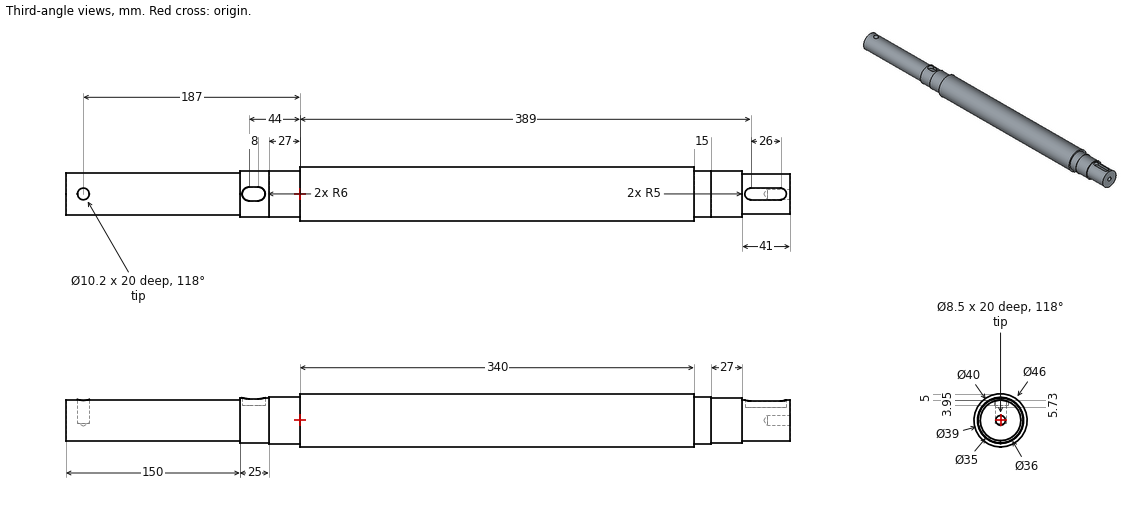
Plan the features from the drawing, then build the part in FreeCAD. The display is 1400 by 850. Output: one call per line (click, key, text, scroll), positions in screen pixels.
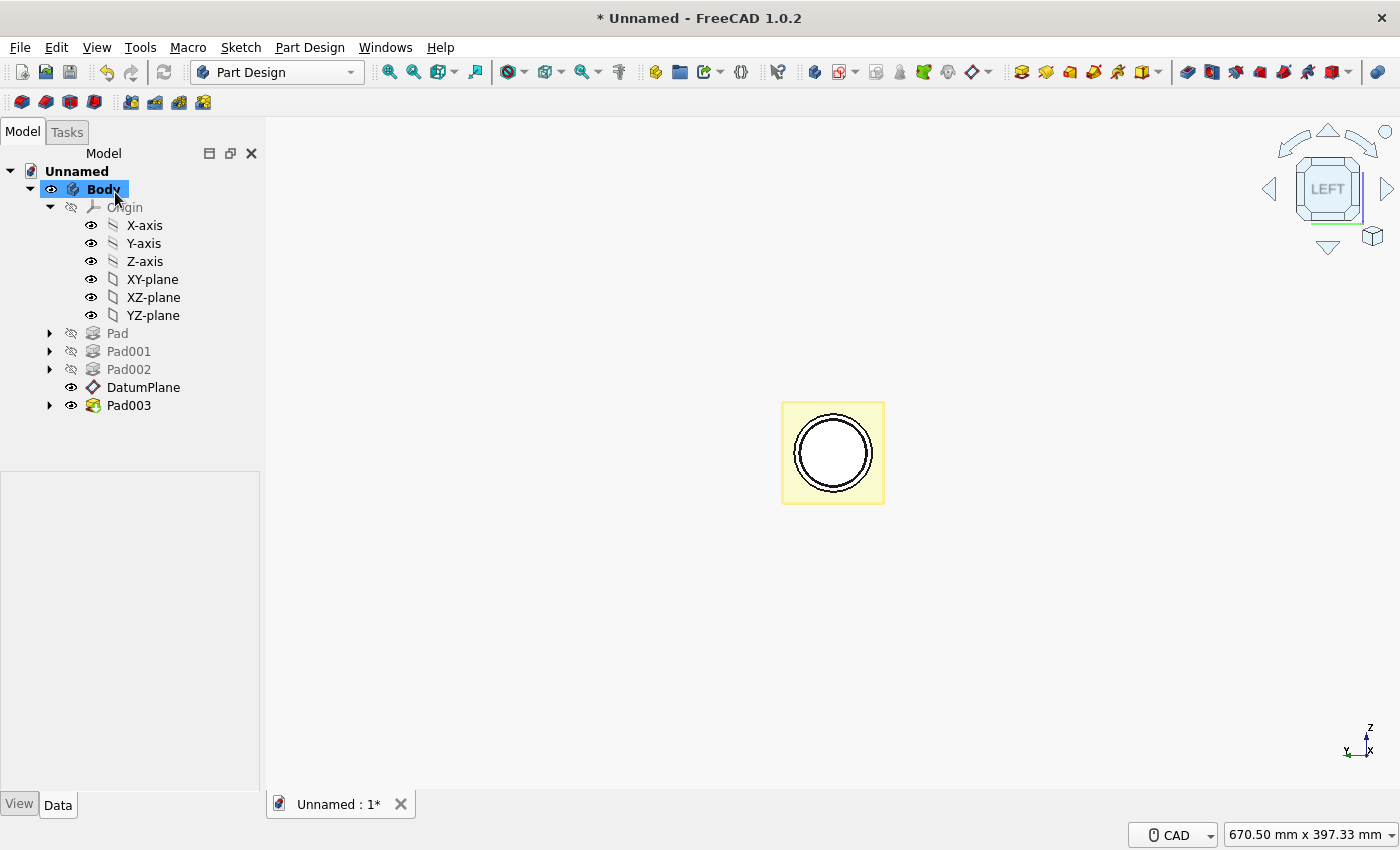
click(116, 387)
key(space)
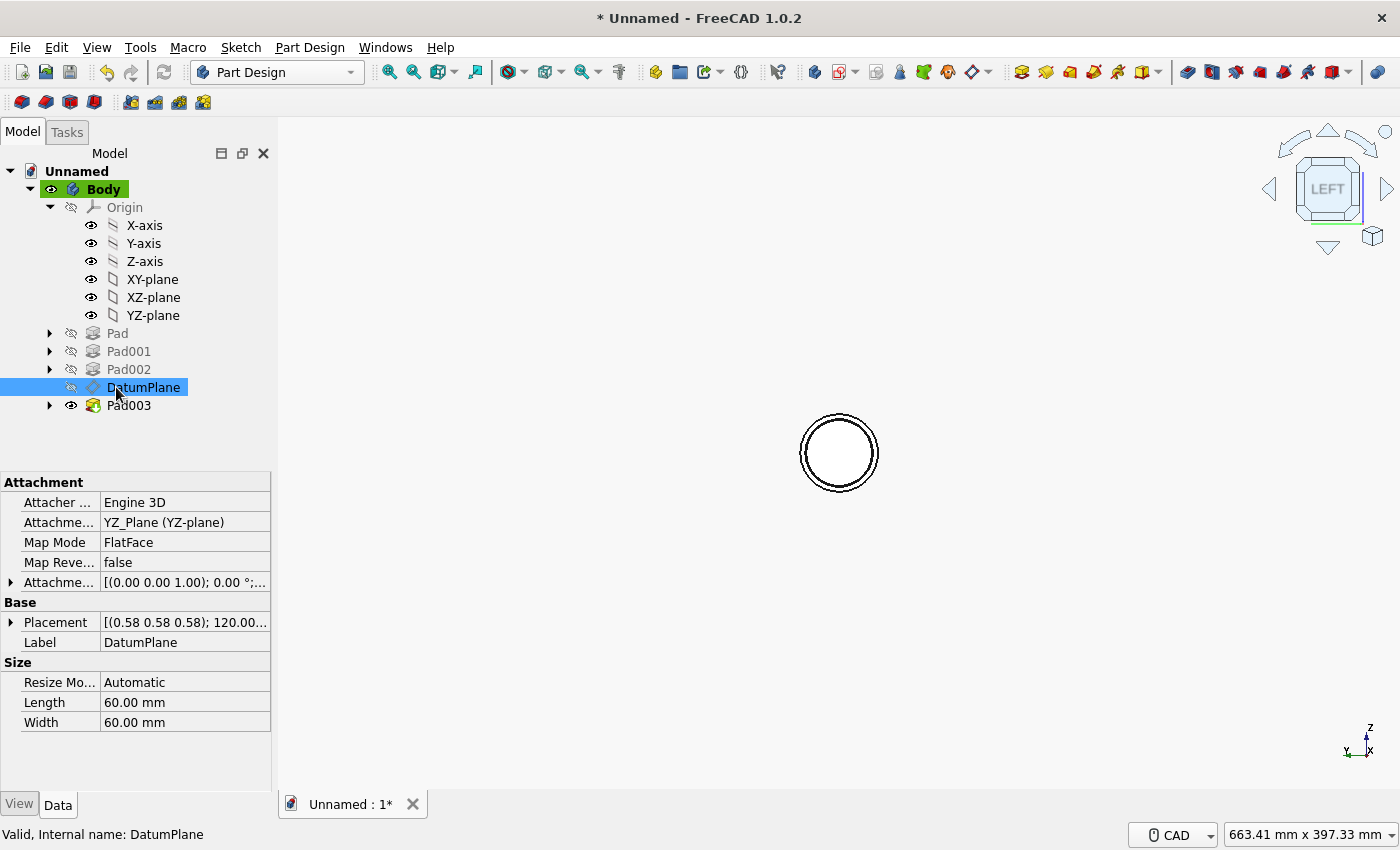
key(v)
key(f)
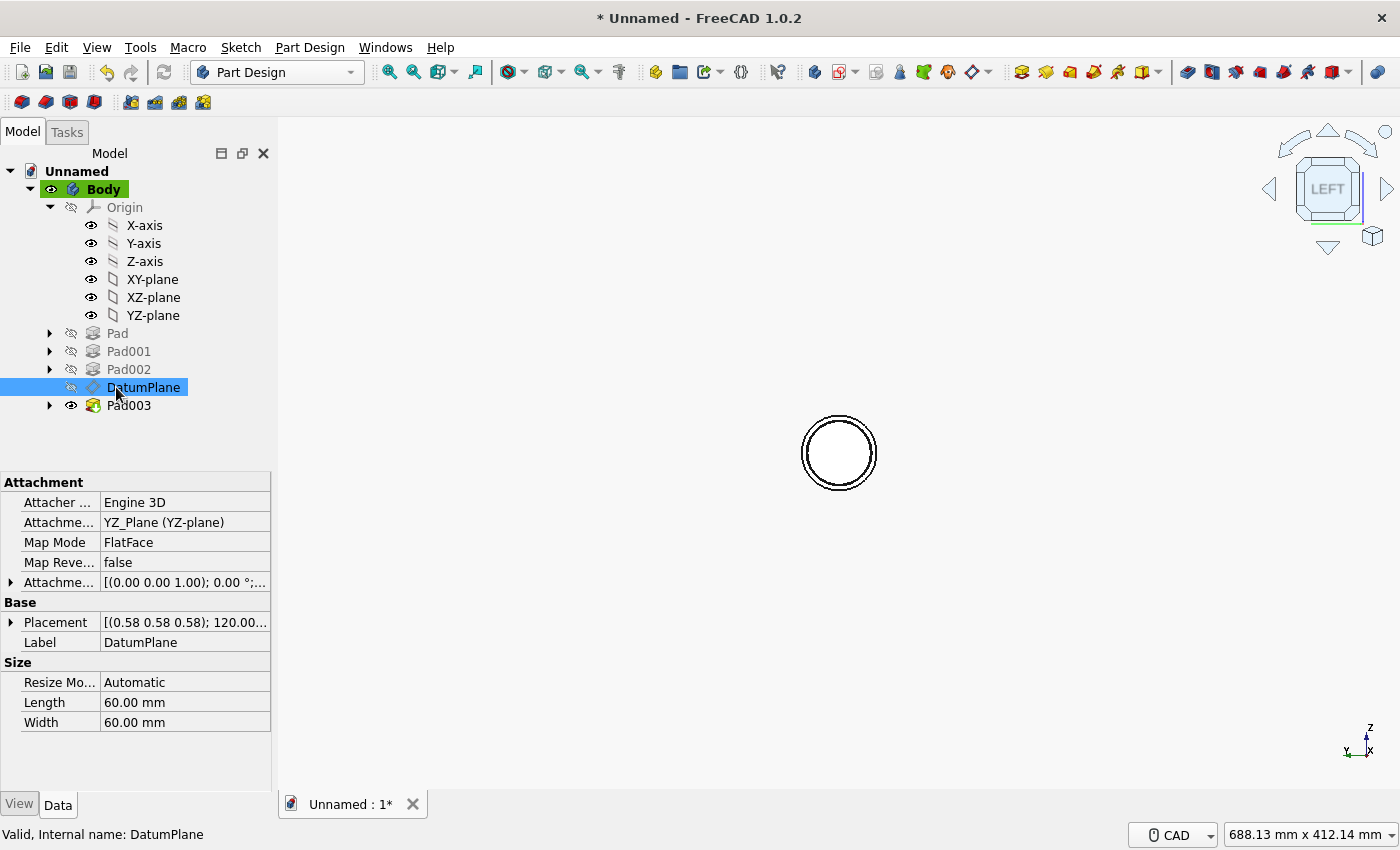
click(136, 315)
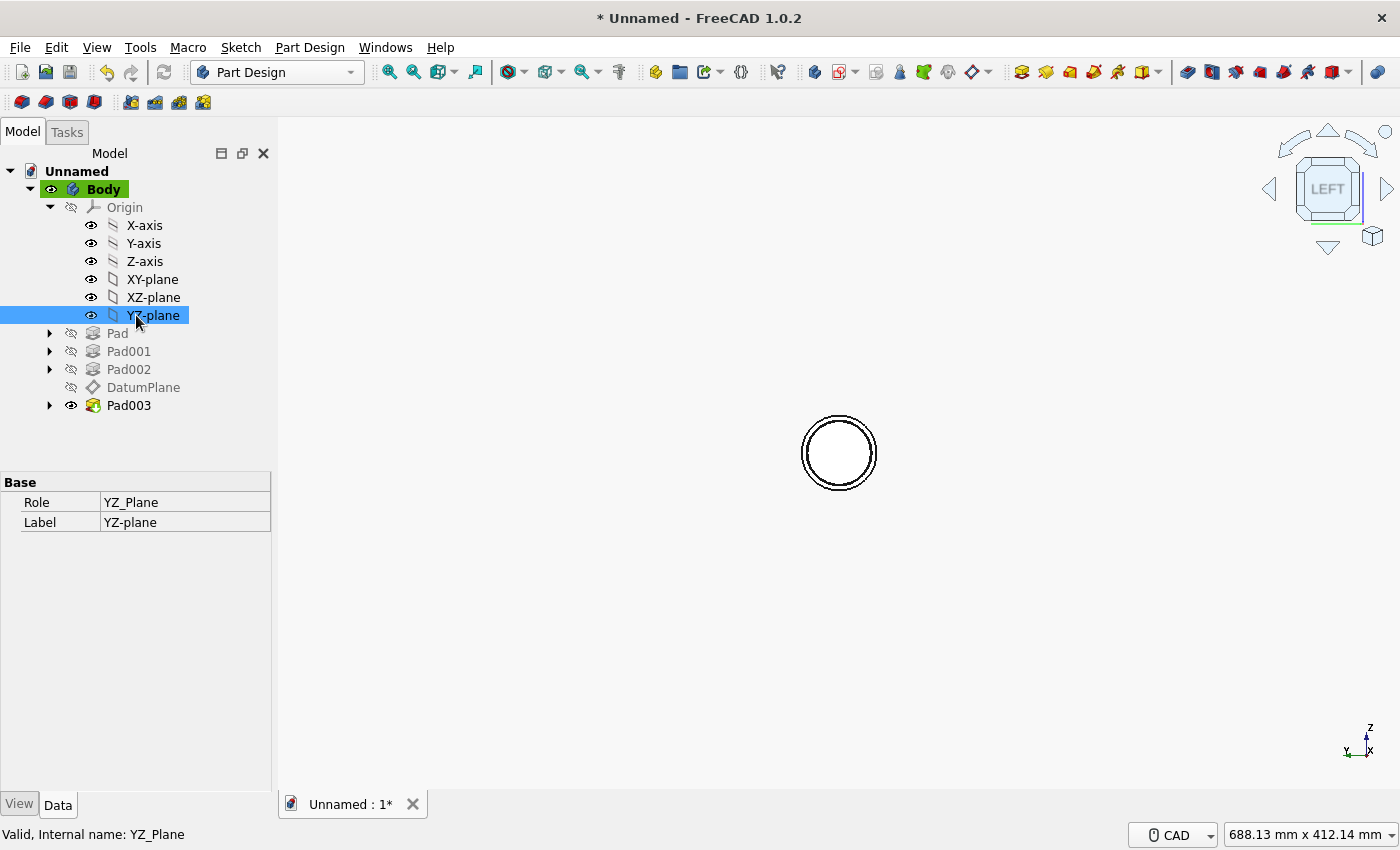
click(972, 72)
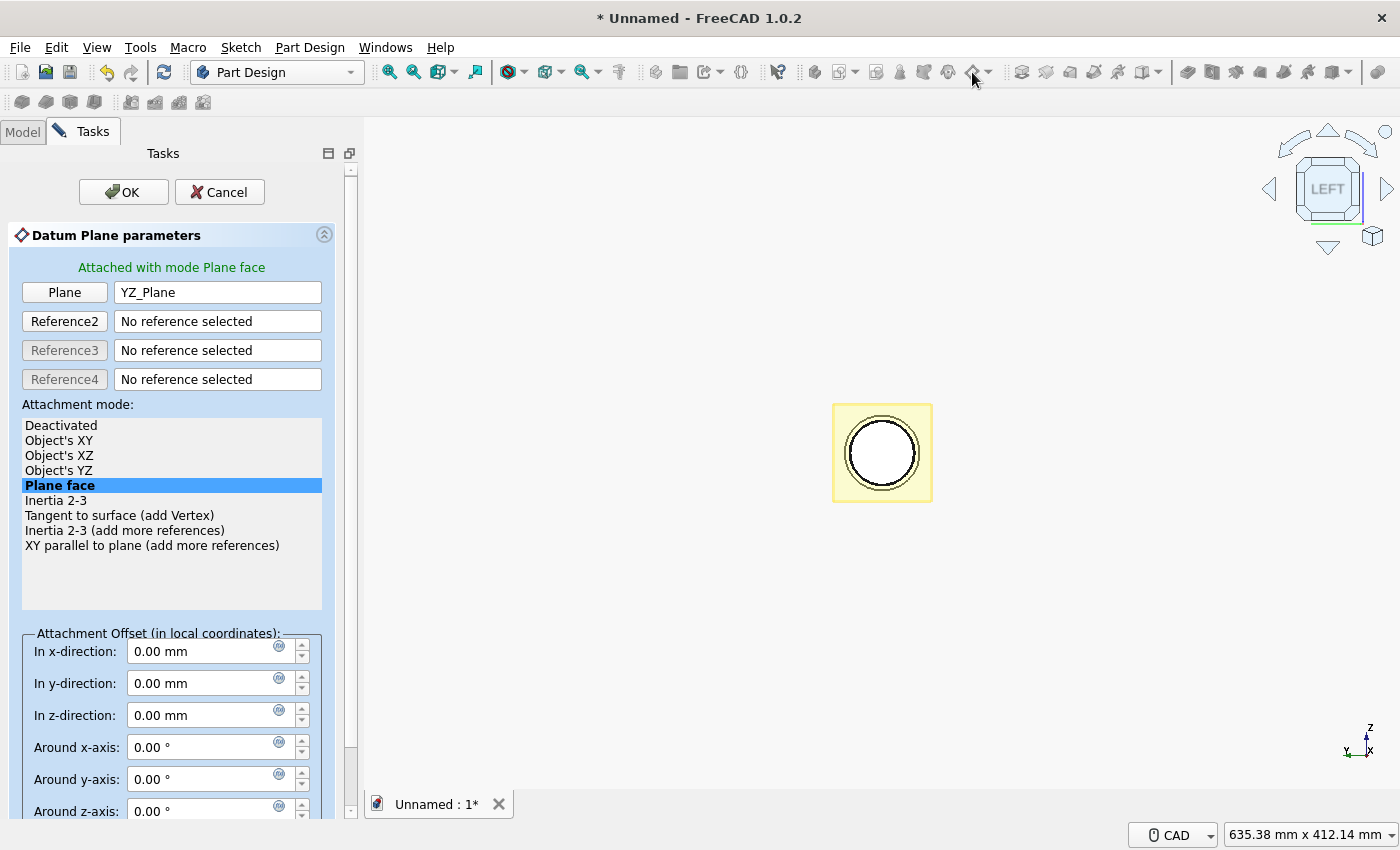
triple_click(210, 715)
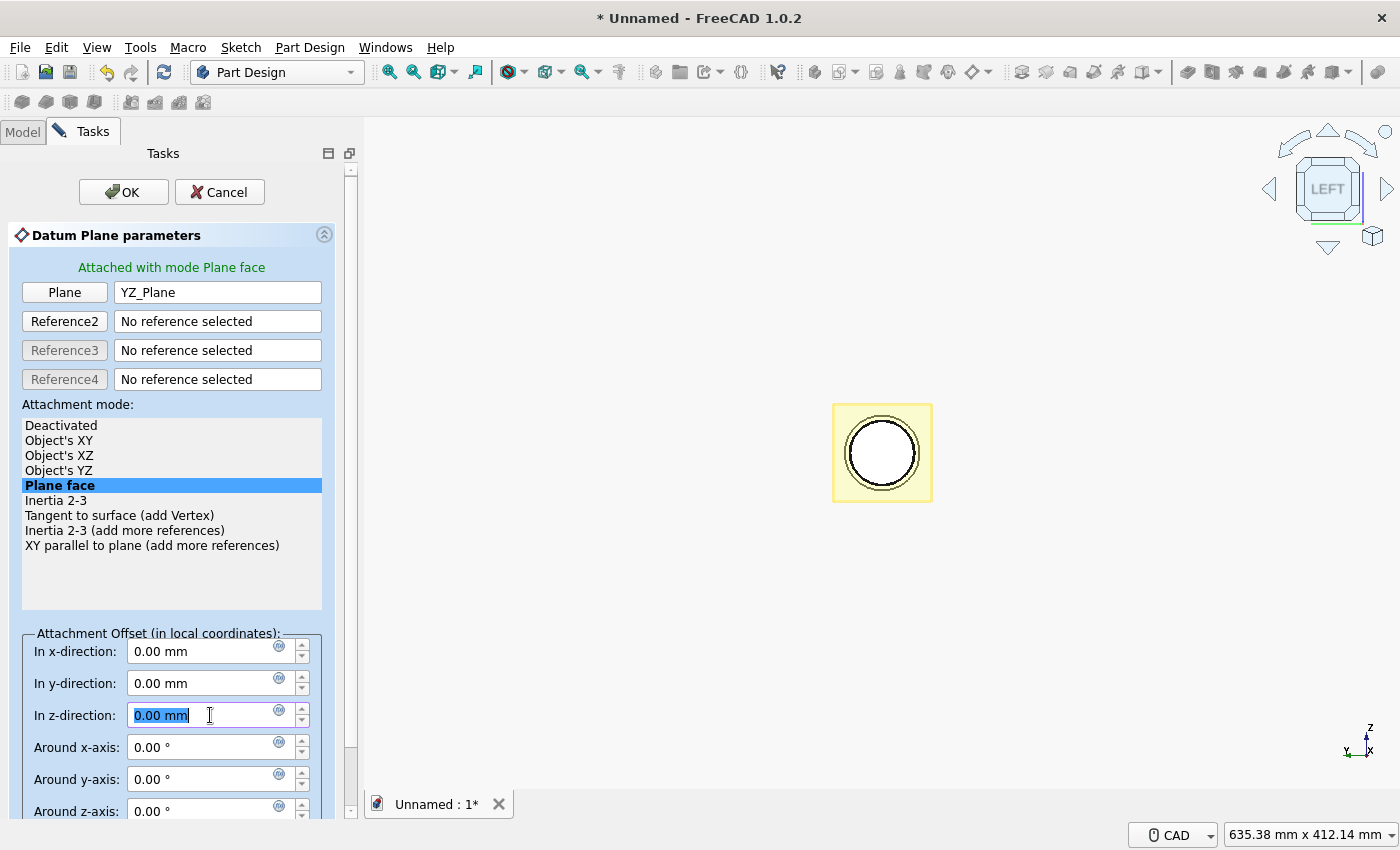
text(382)
key(Tab)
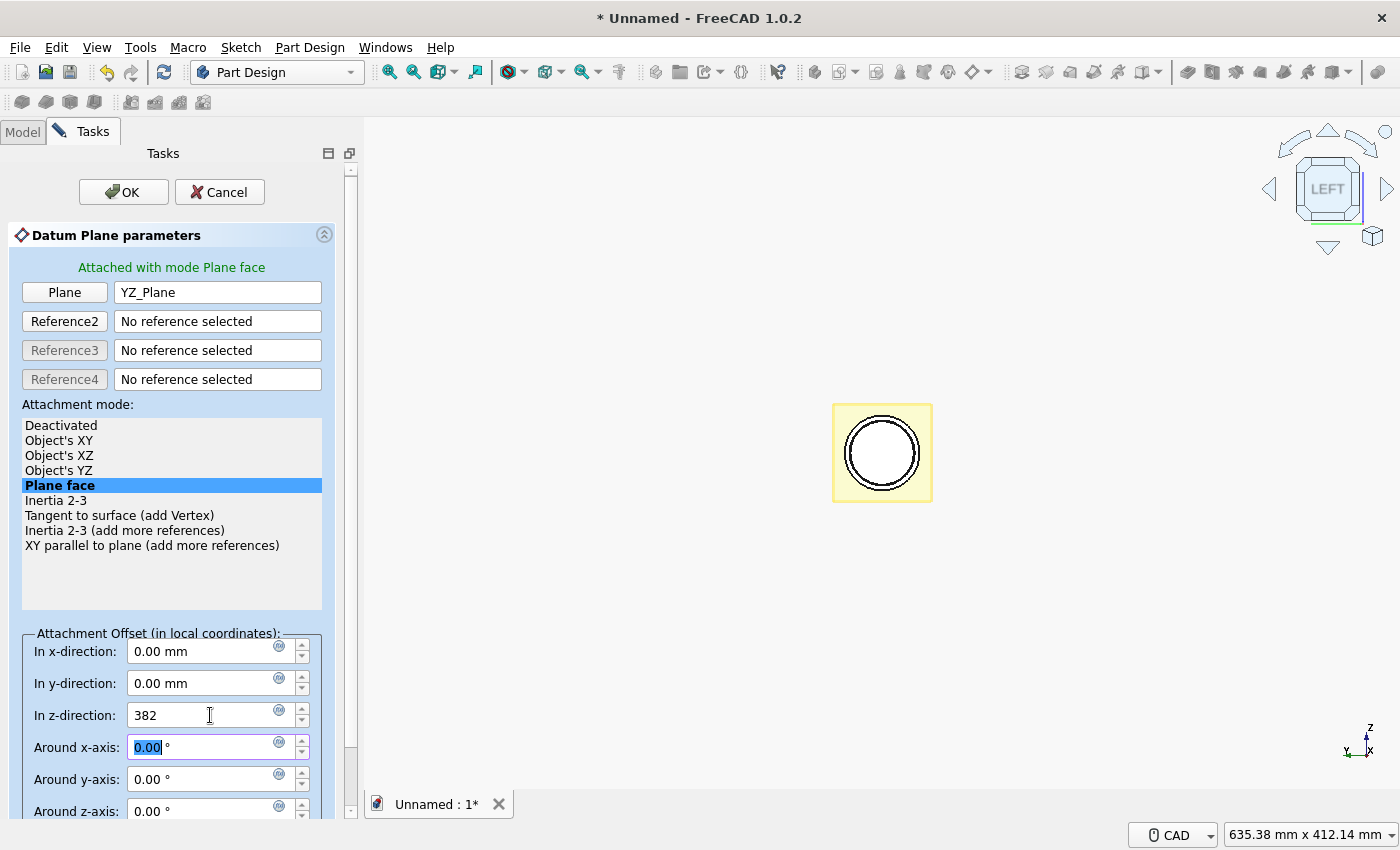
click(124, 192)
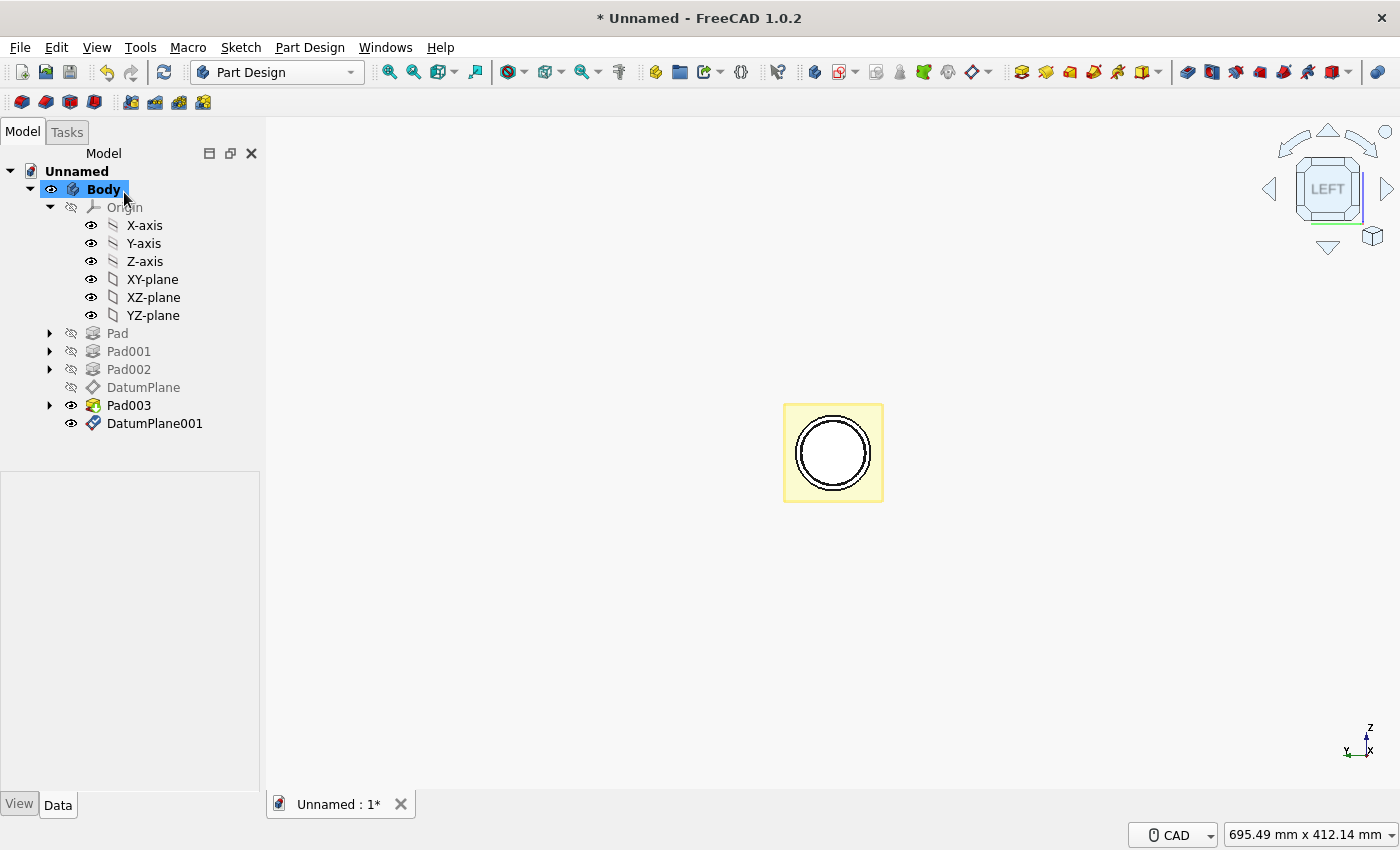
click(116, 423)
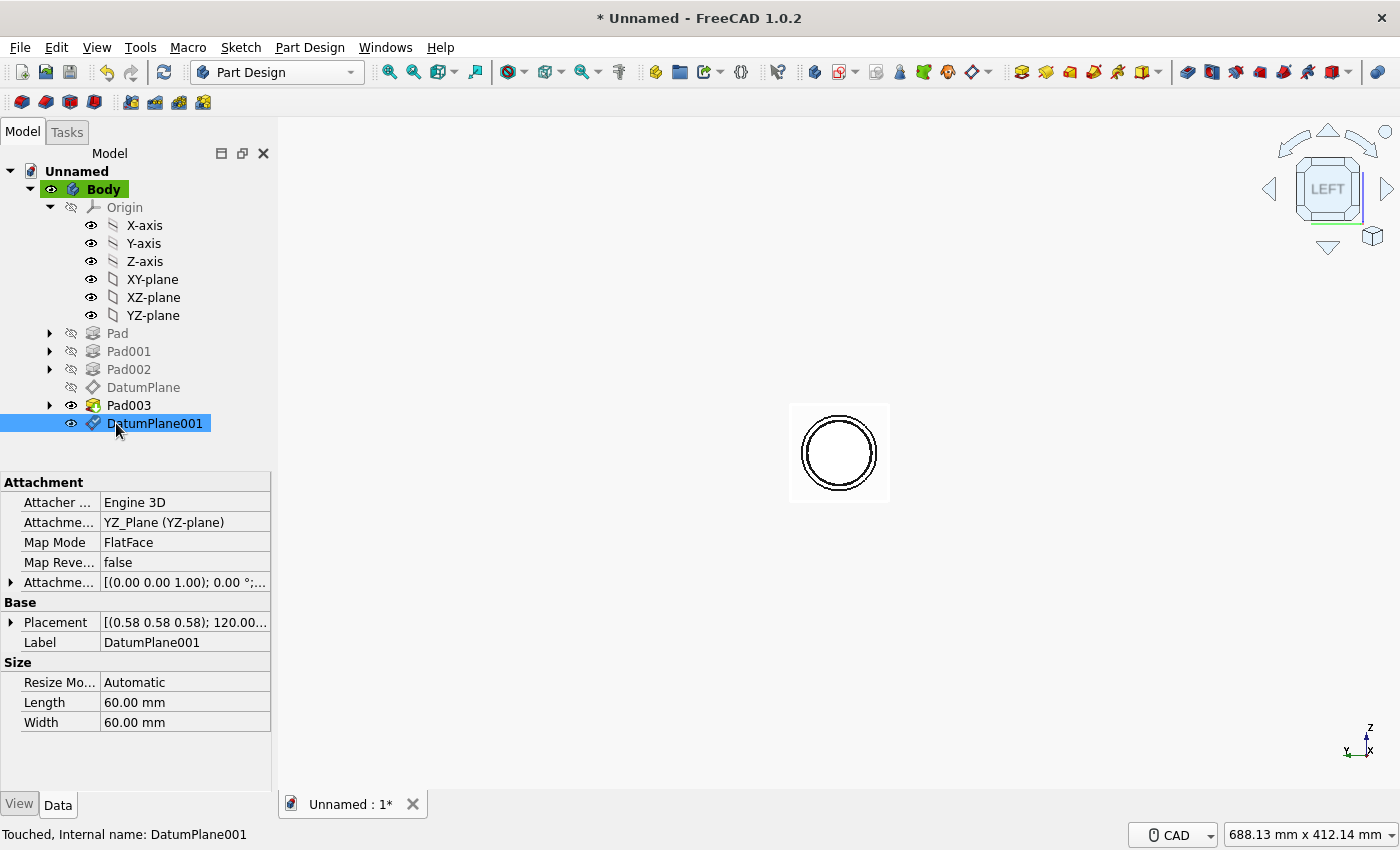
click(840, 72)